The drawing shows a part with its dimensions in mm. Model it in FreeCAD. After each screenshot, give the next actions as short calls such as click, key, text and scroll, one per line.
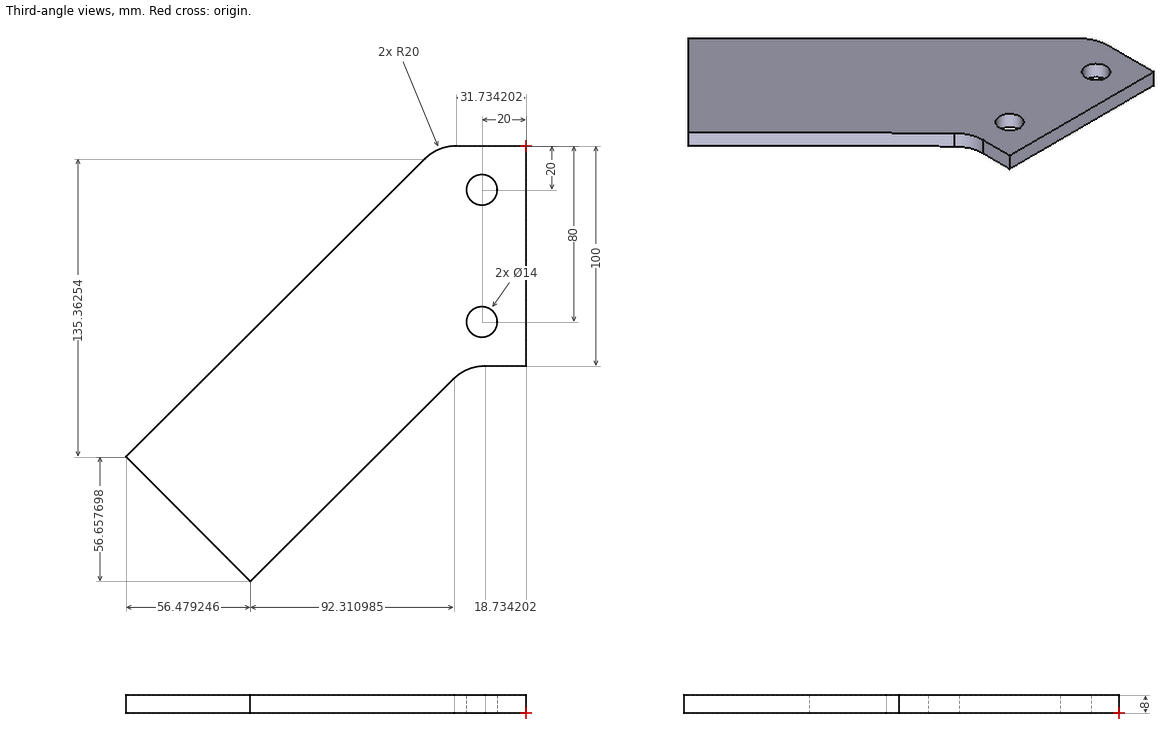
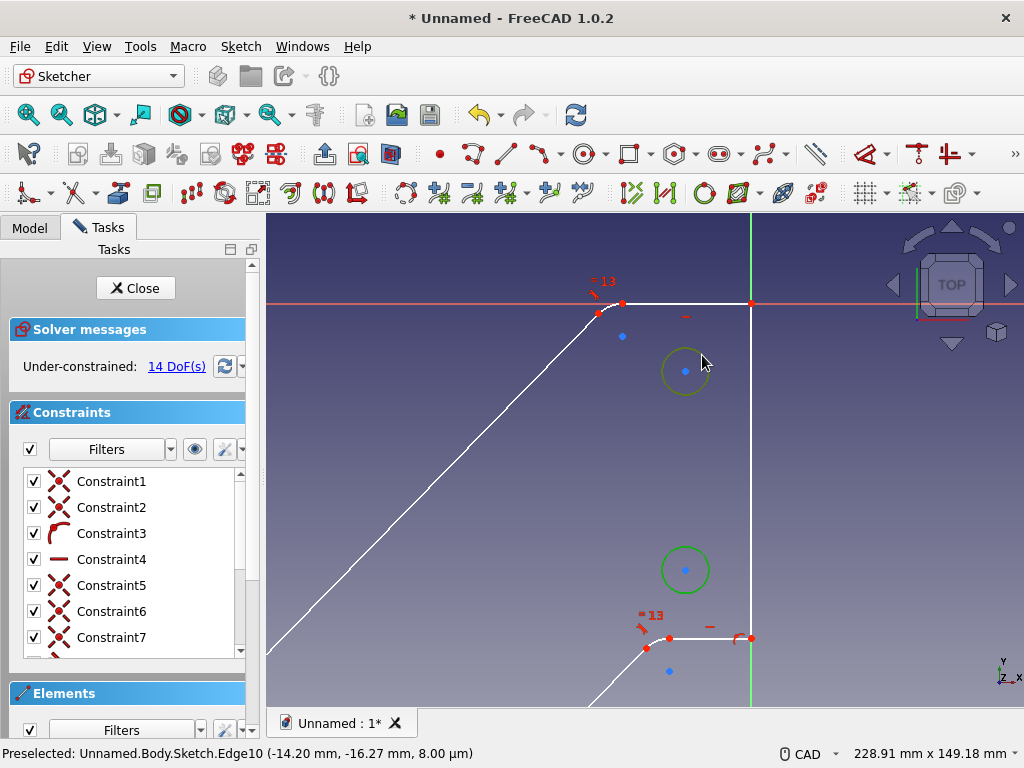
key(e)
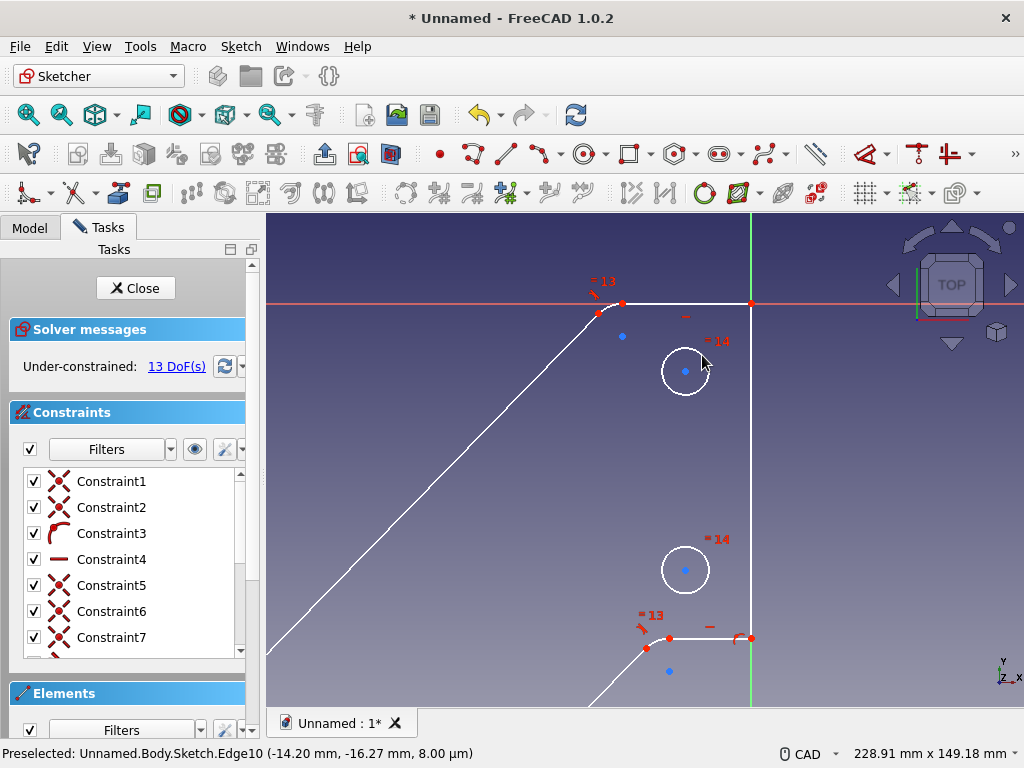
click(864, 154)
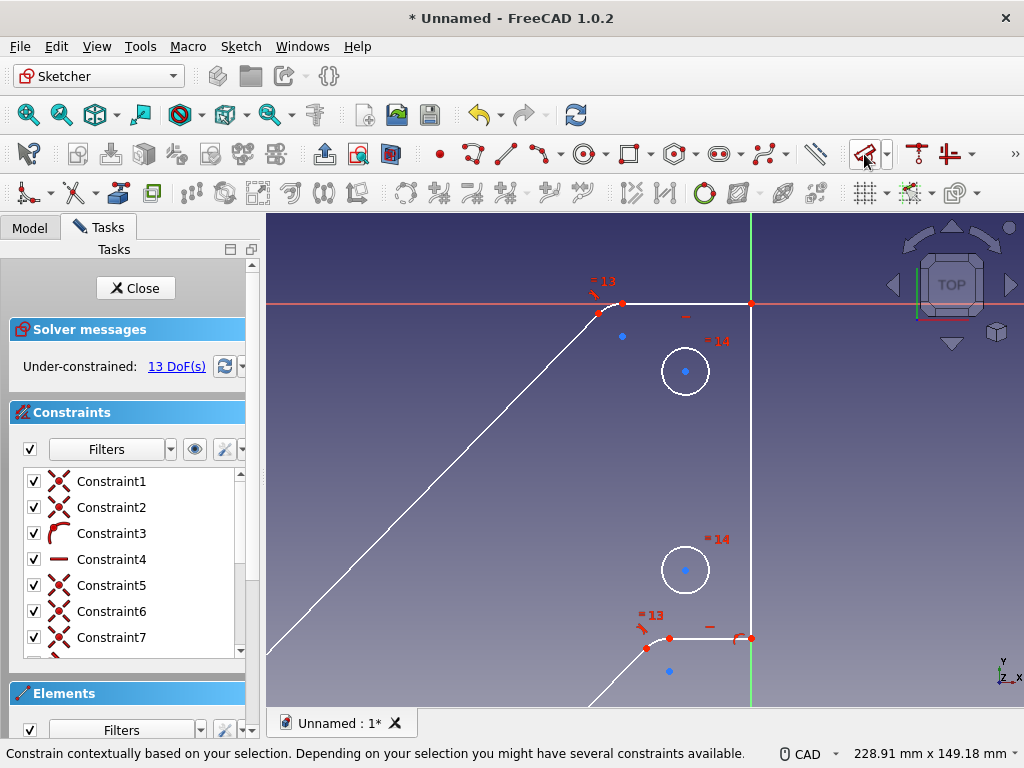
click(657, 641)
click(645, 611)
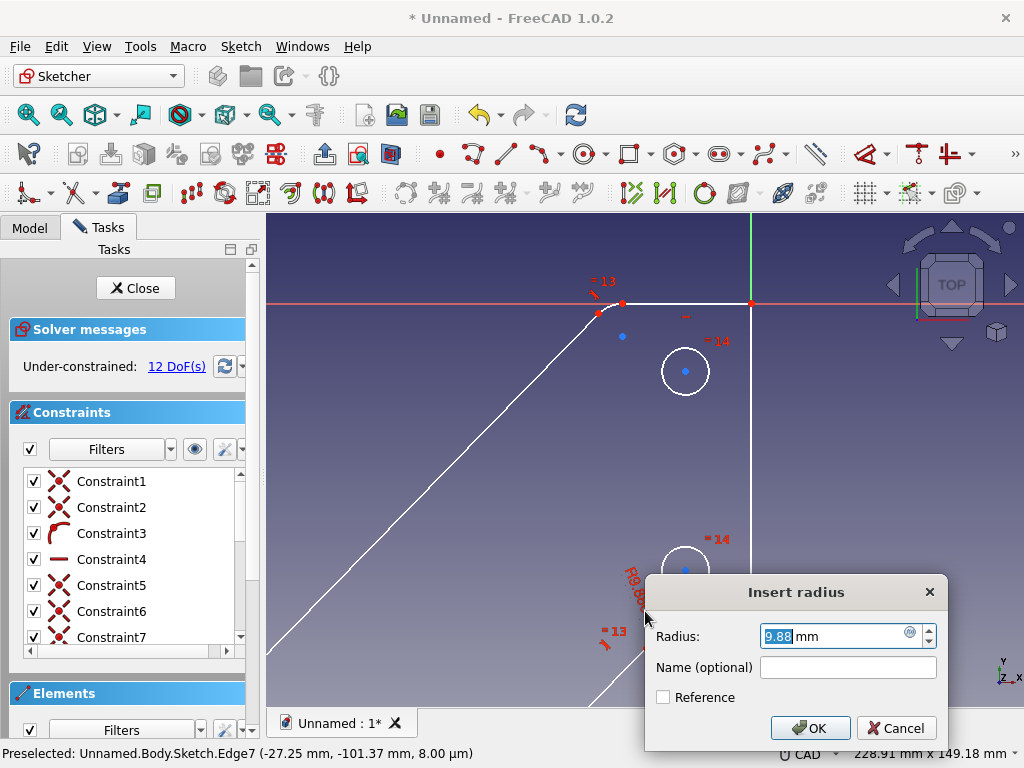
text(20)
key(Return)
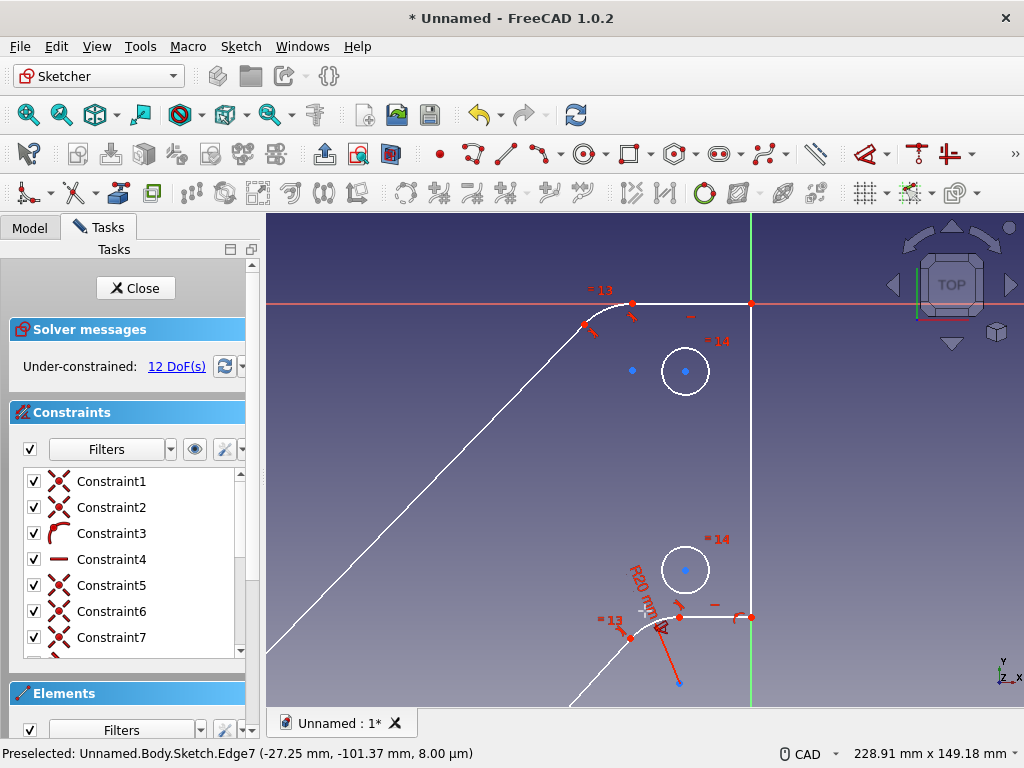
click(702, 553)
click(724, 530)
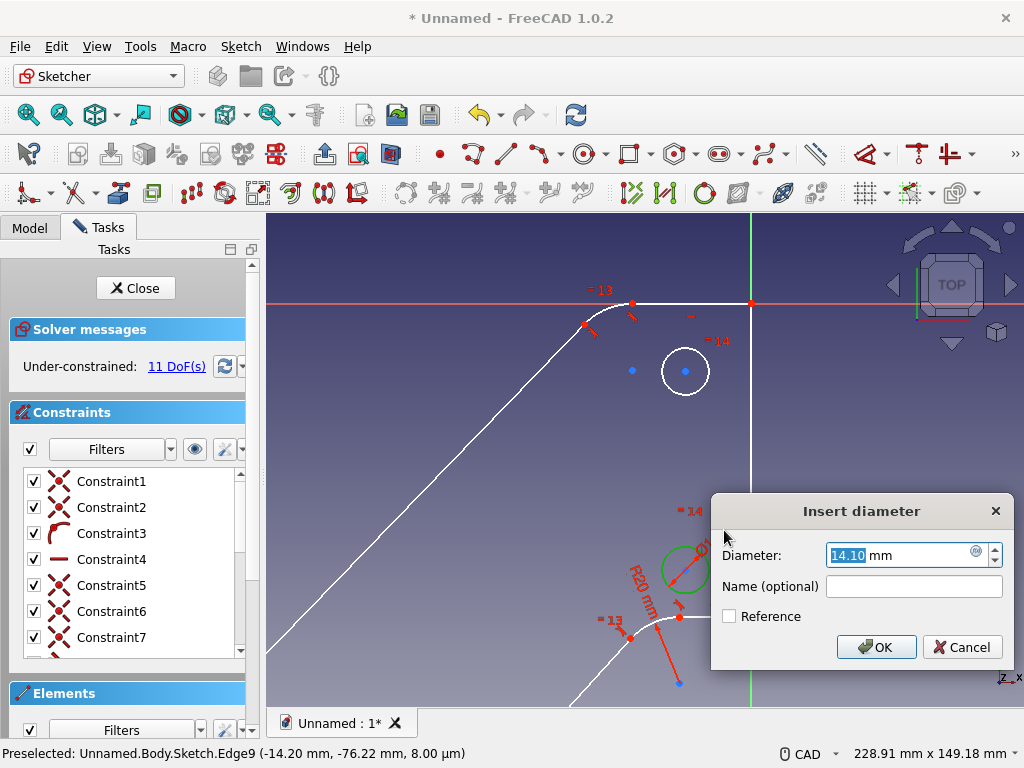
text(14)
key(Return)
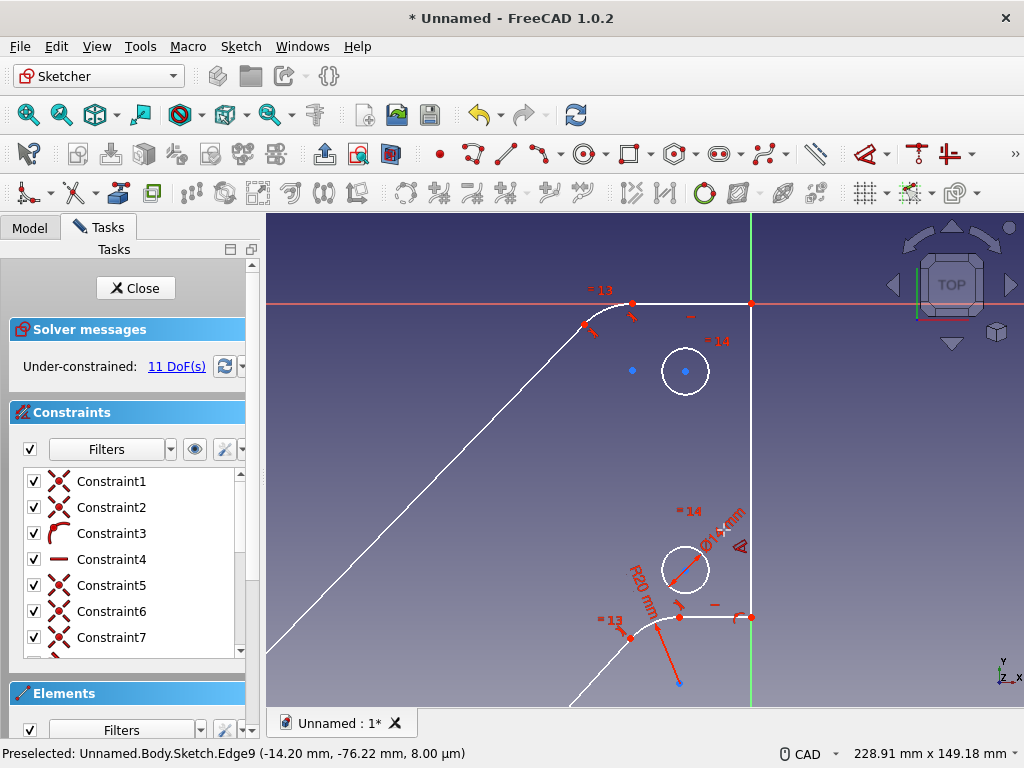
click(685, 570)
click(718, 270)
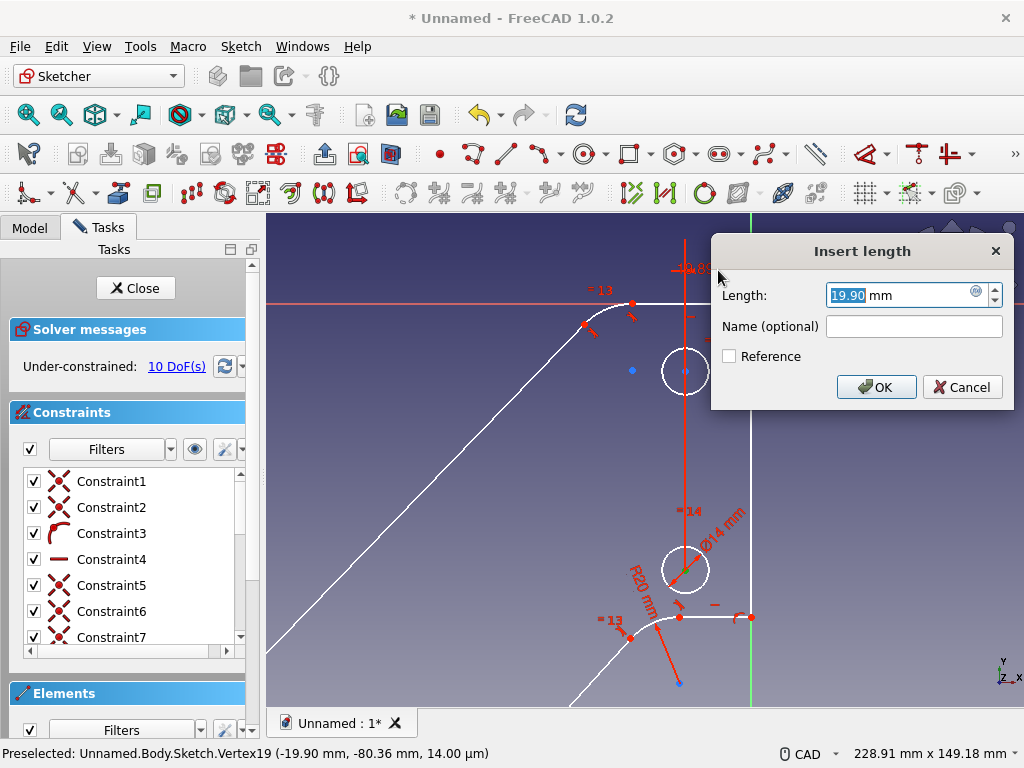
text(20)
key(Return)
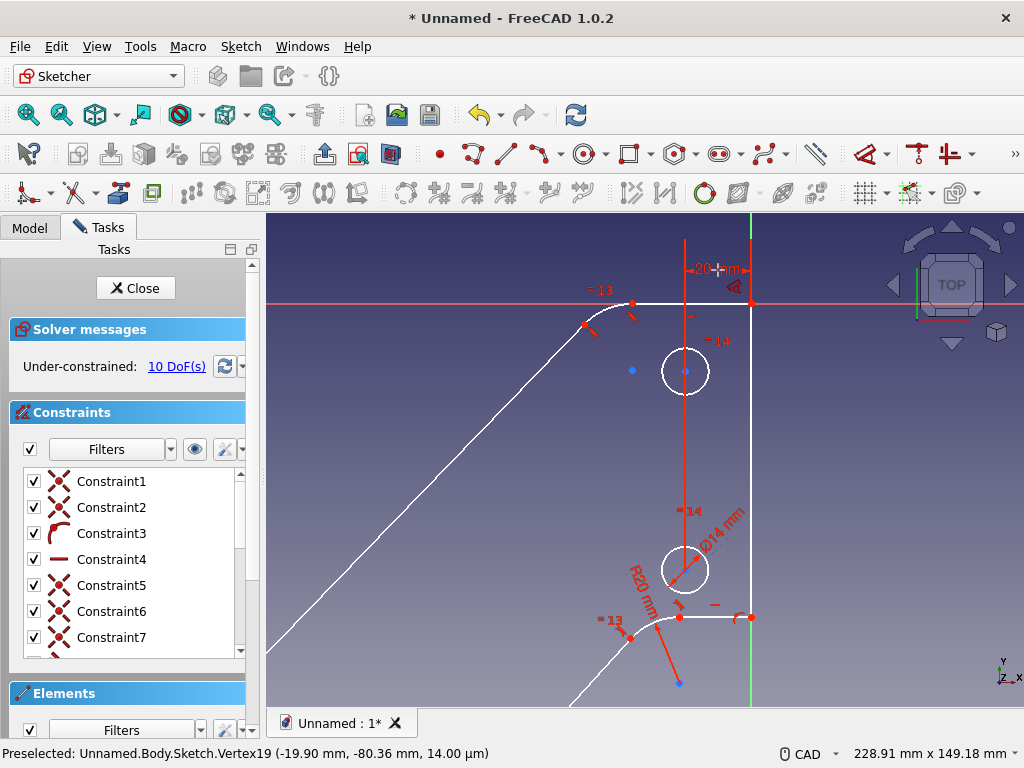
click(685, 570)
click(785, 437)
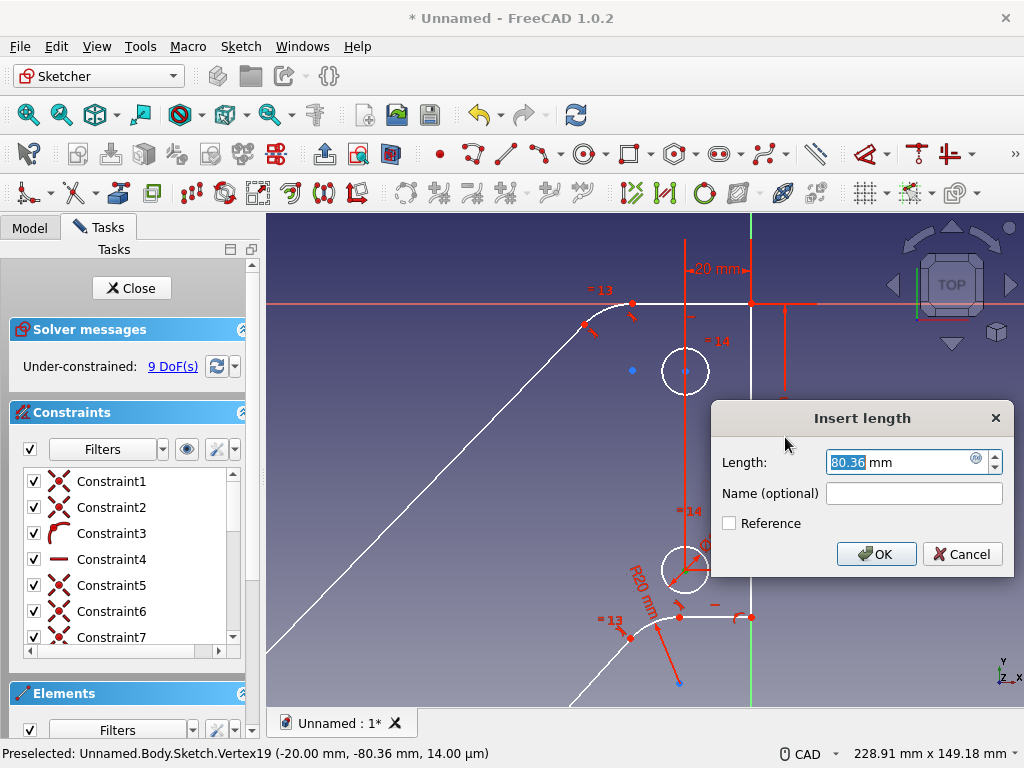
text(80)
key(Return)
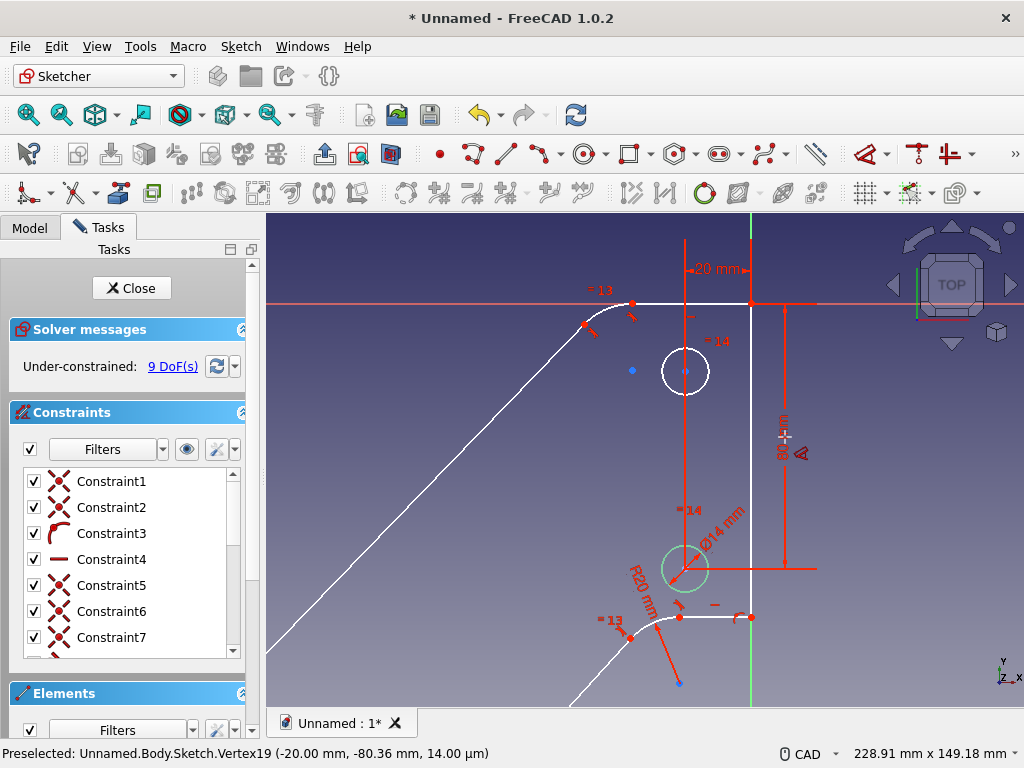
click(685, 372)
click(718, 406)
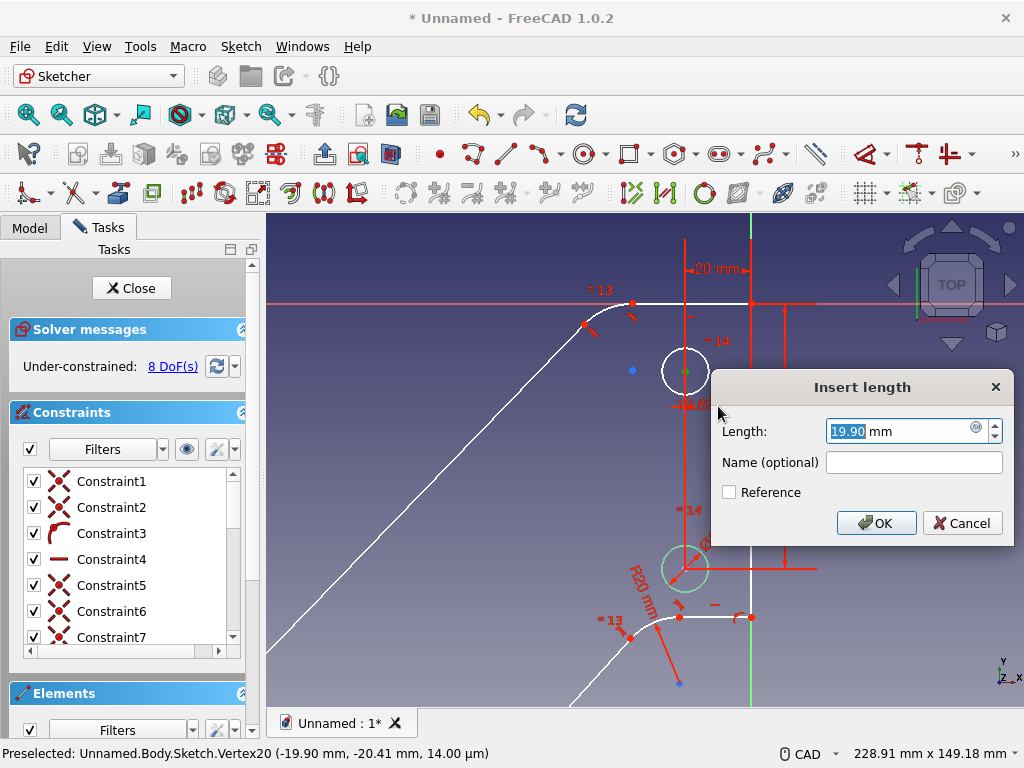
text(20)
key(Return)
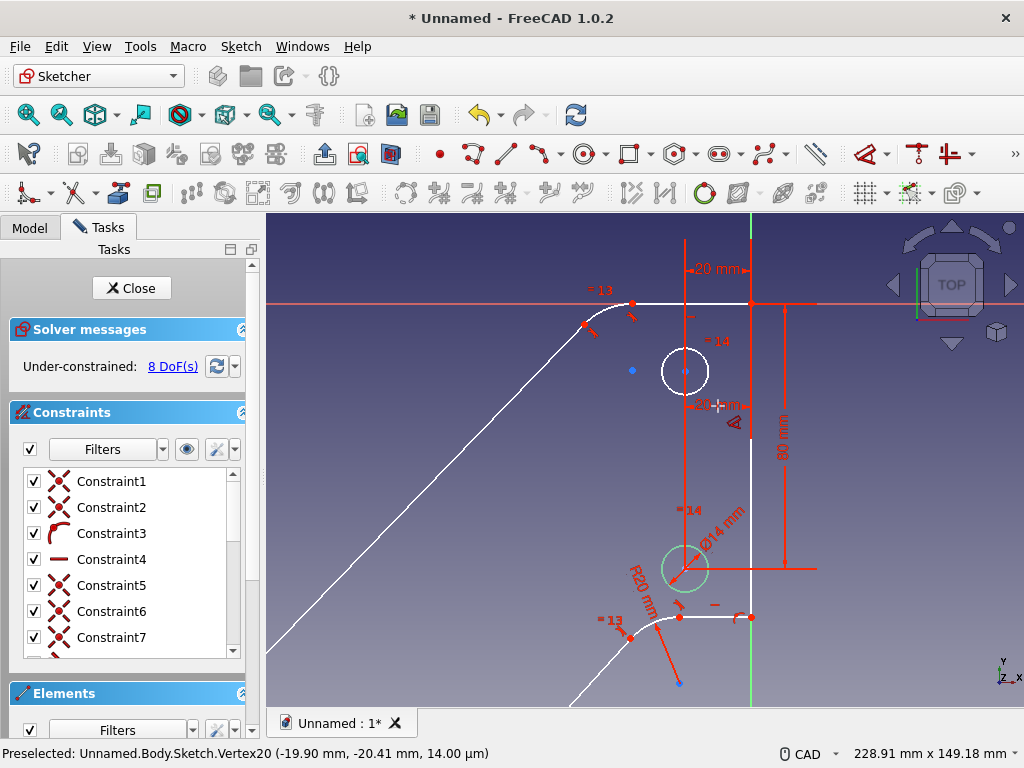
click(685, 372)
click(785, 338)